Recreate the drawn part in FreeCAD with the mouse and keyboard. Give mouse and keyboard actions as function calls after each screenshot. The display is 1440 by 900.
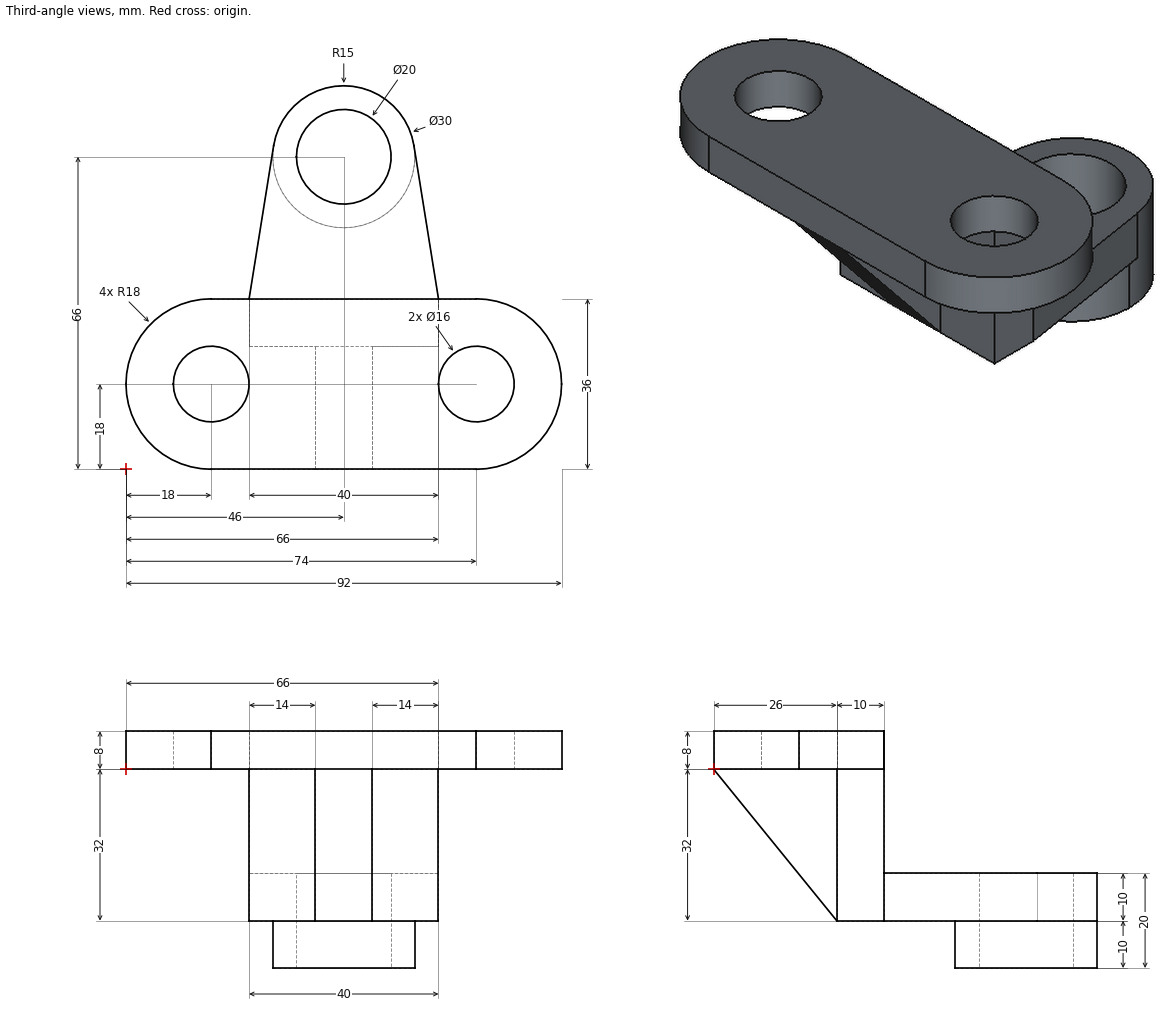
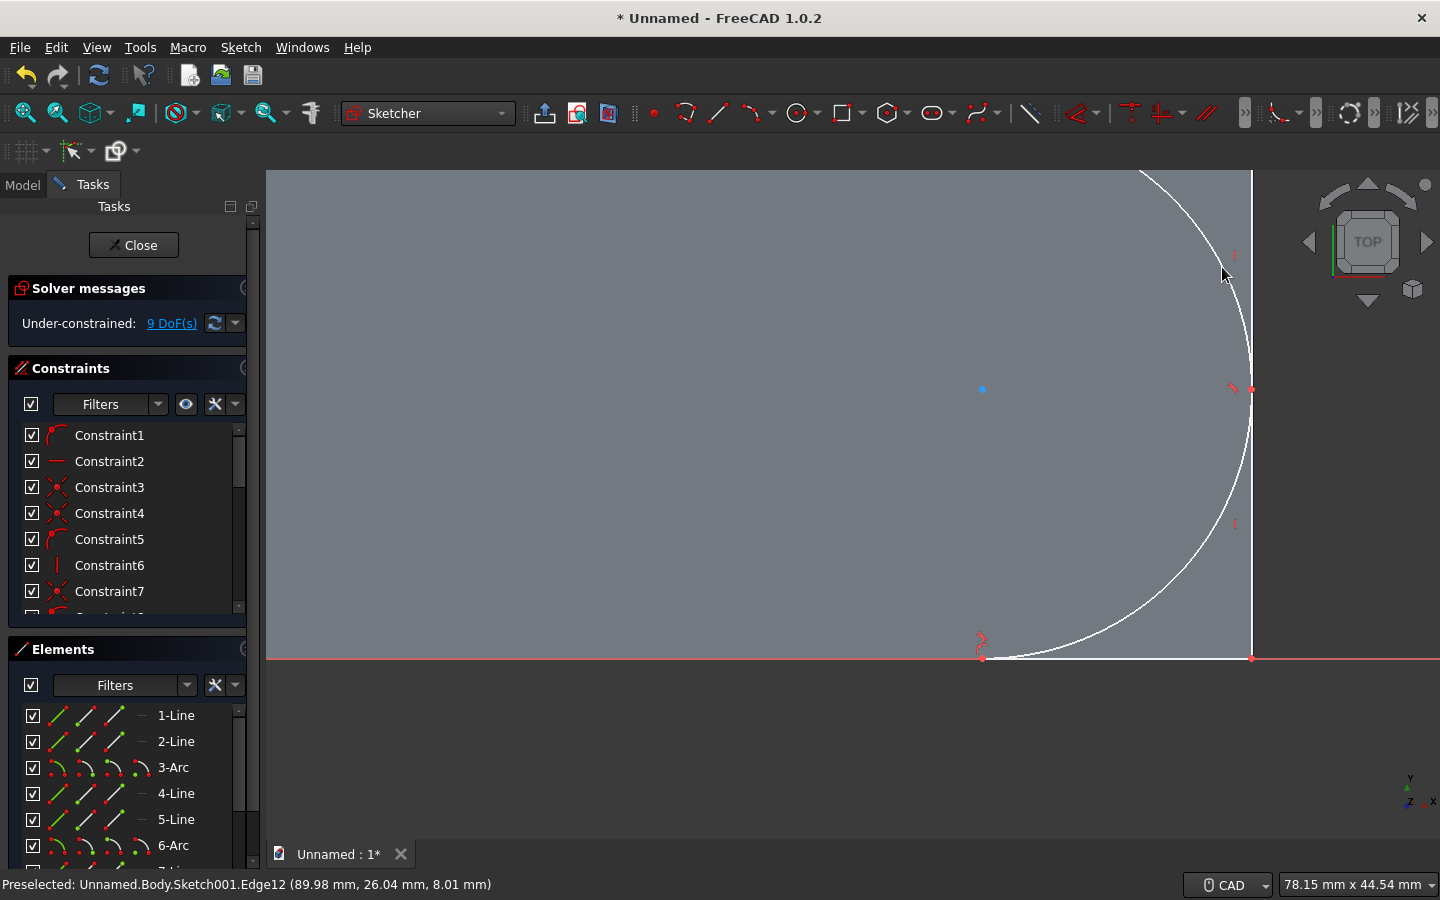
scroll(1055, 646, down, 3)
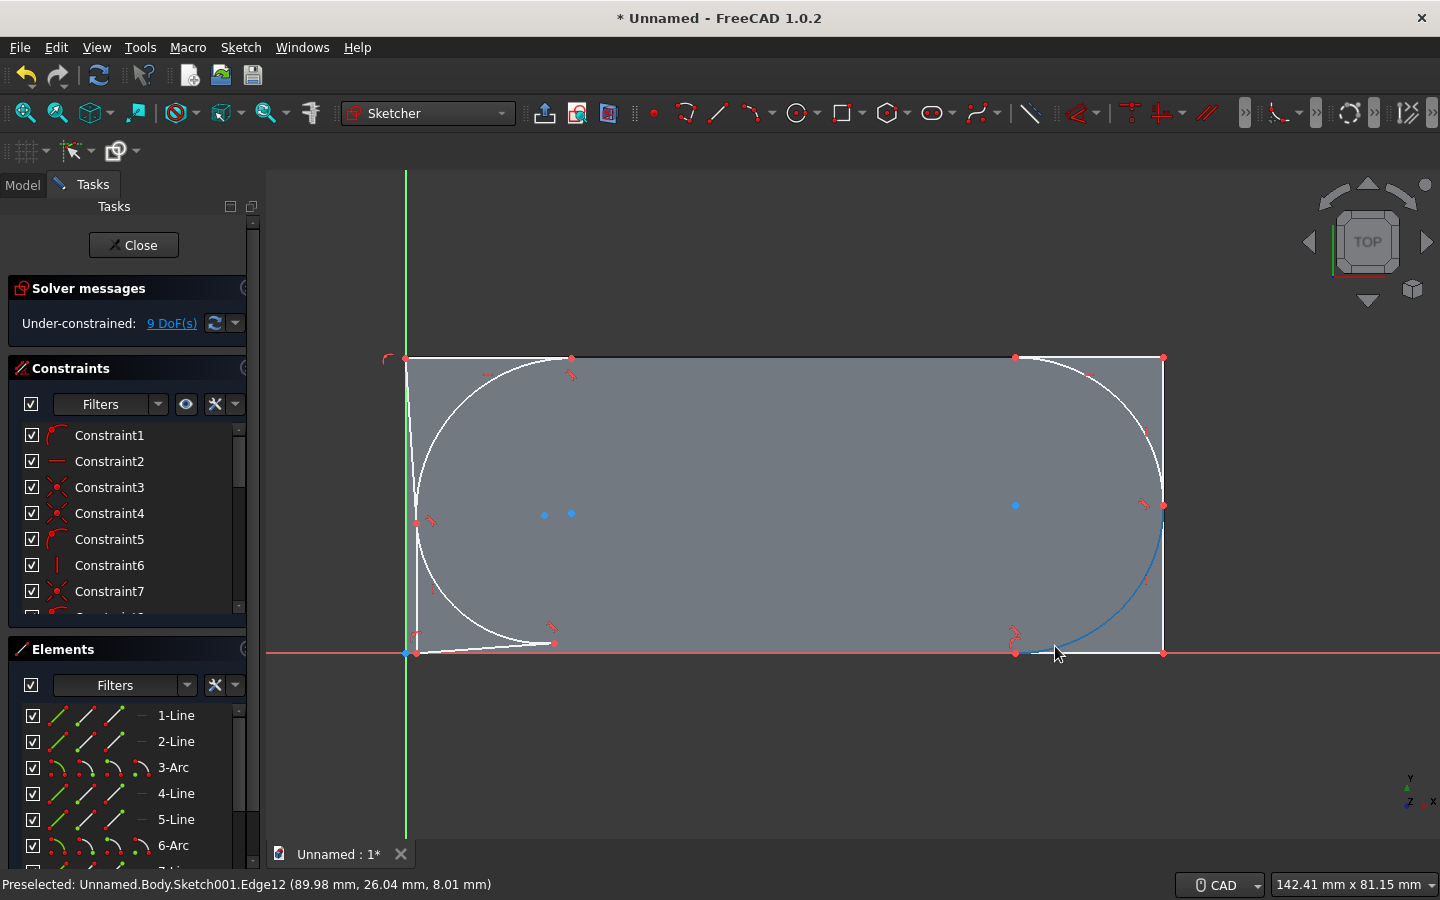
click(1119, 357)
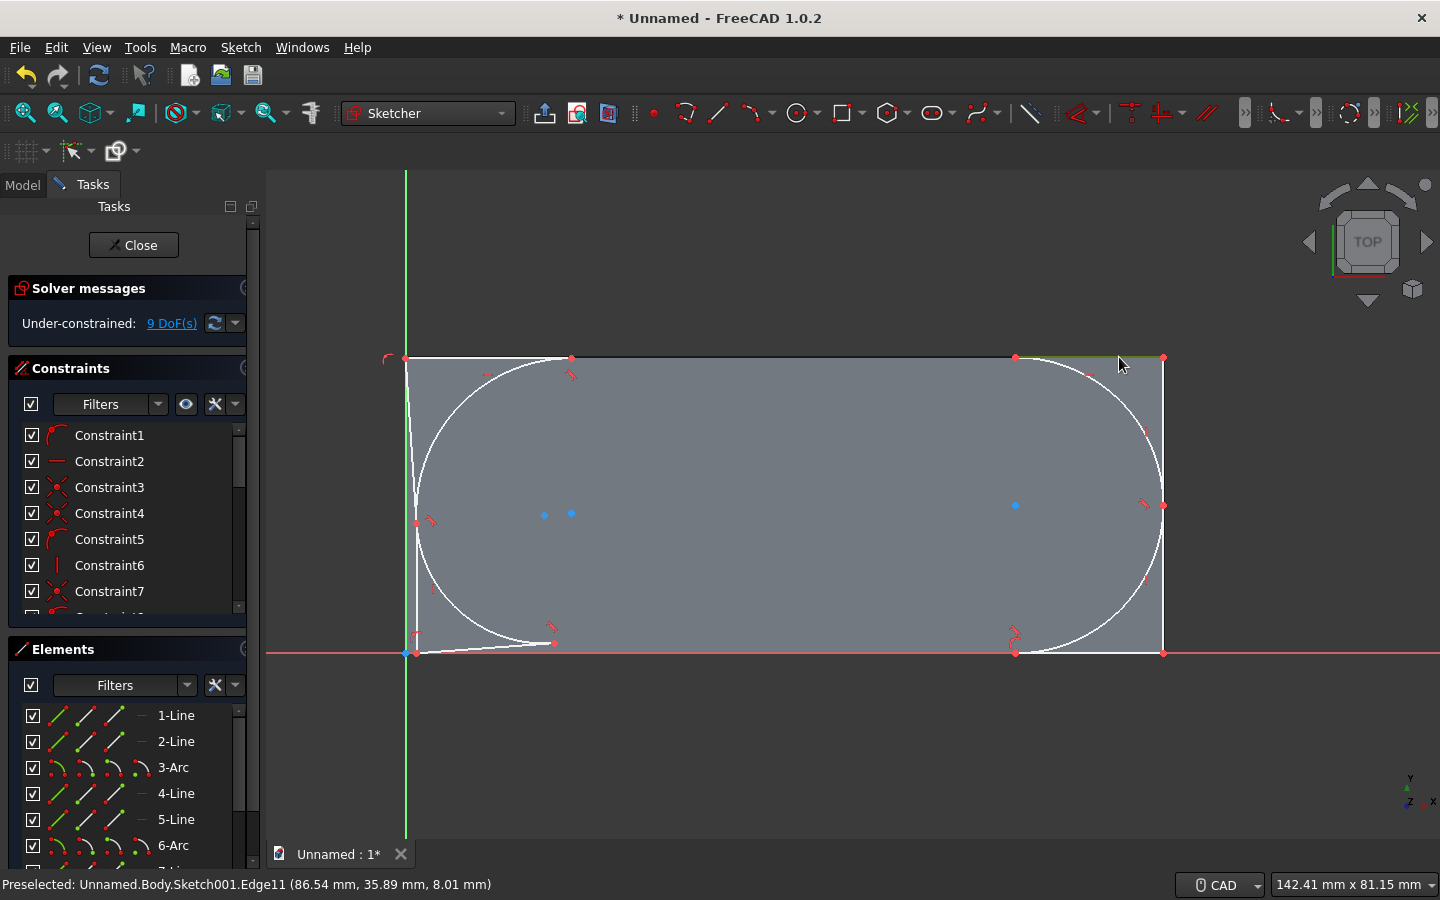
click(1147, 438)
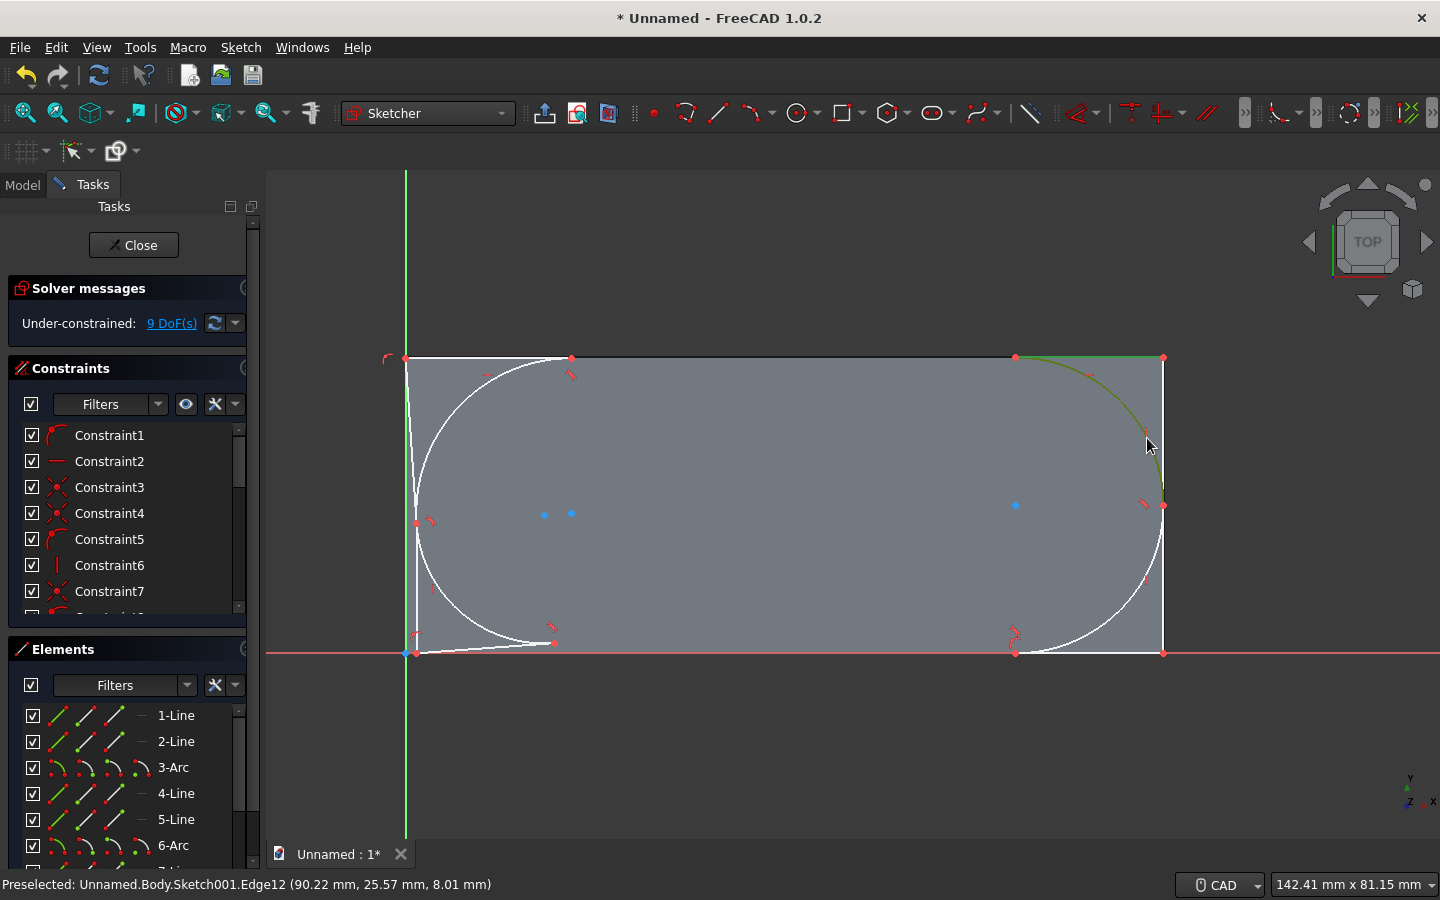
key(t)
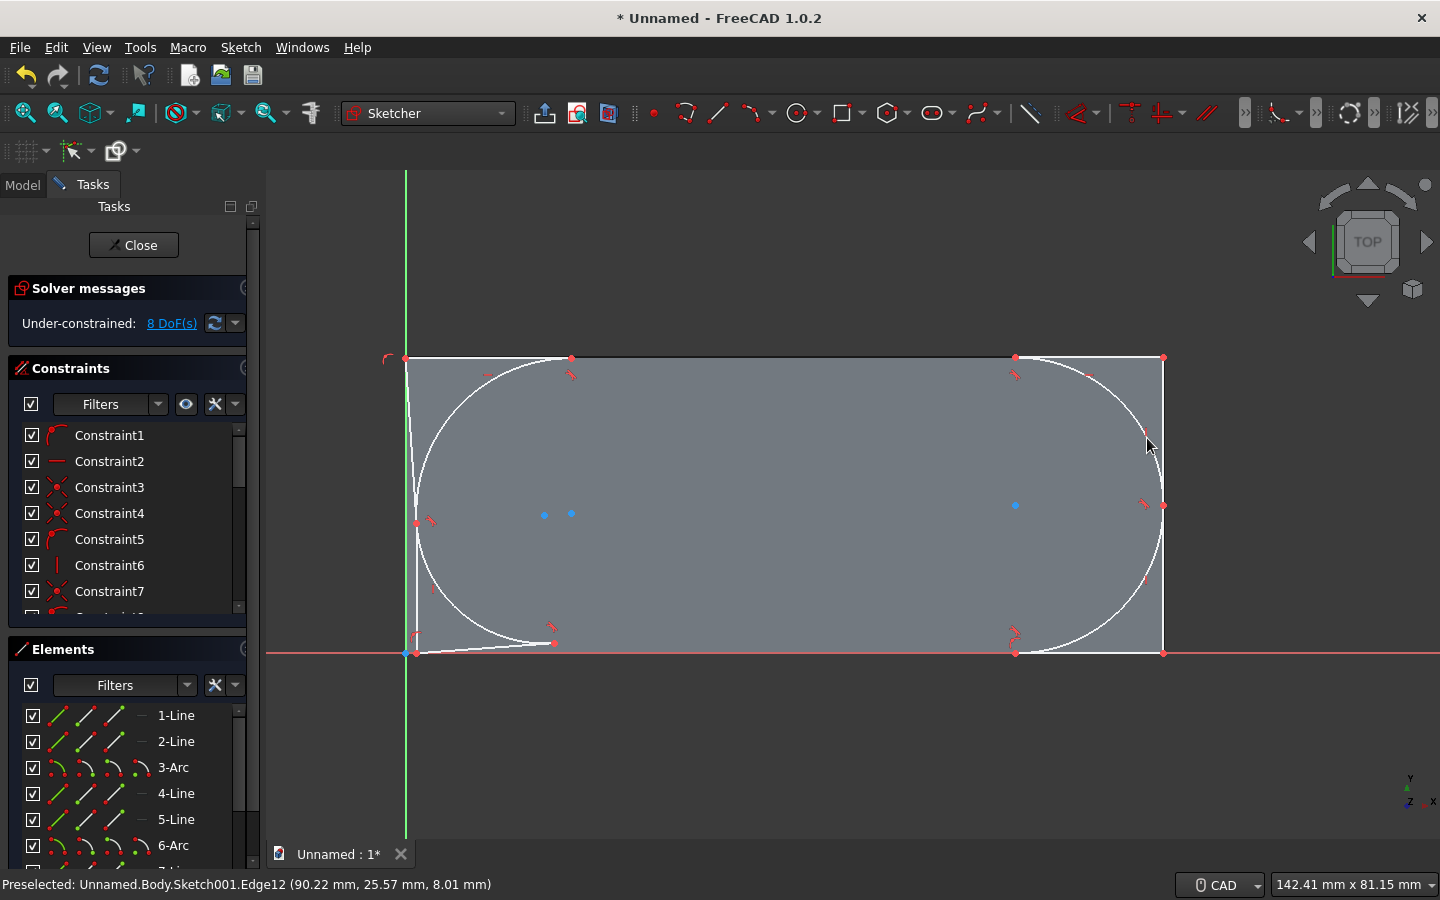
click(409, 408)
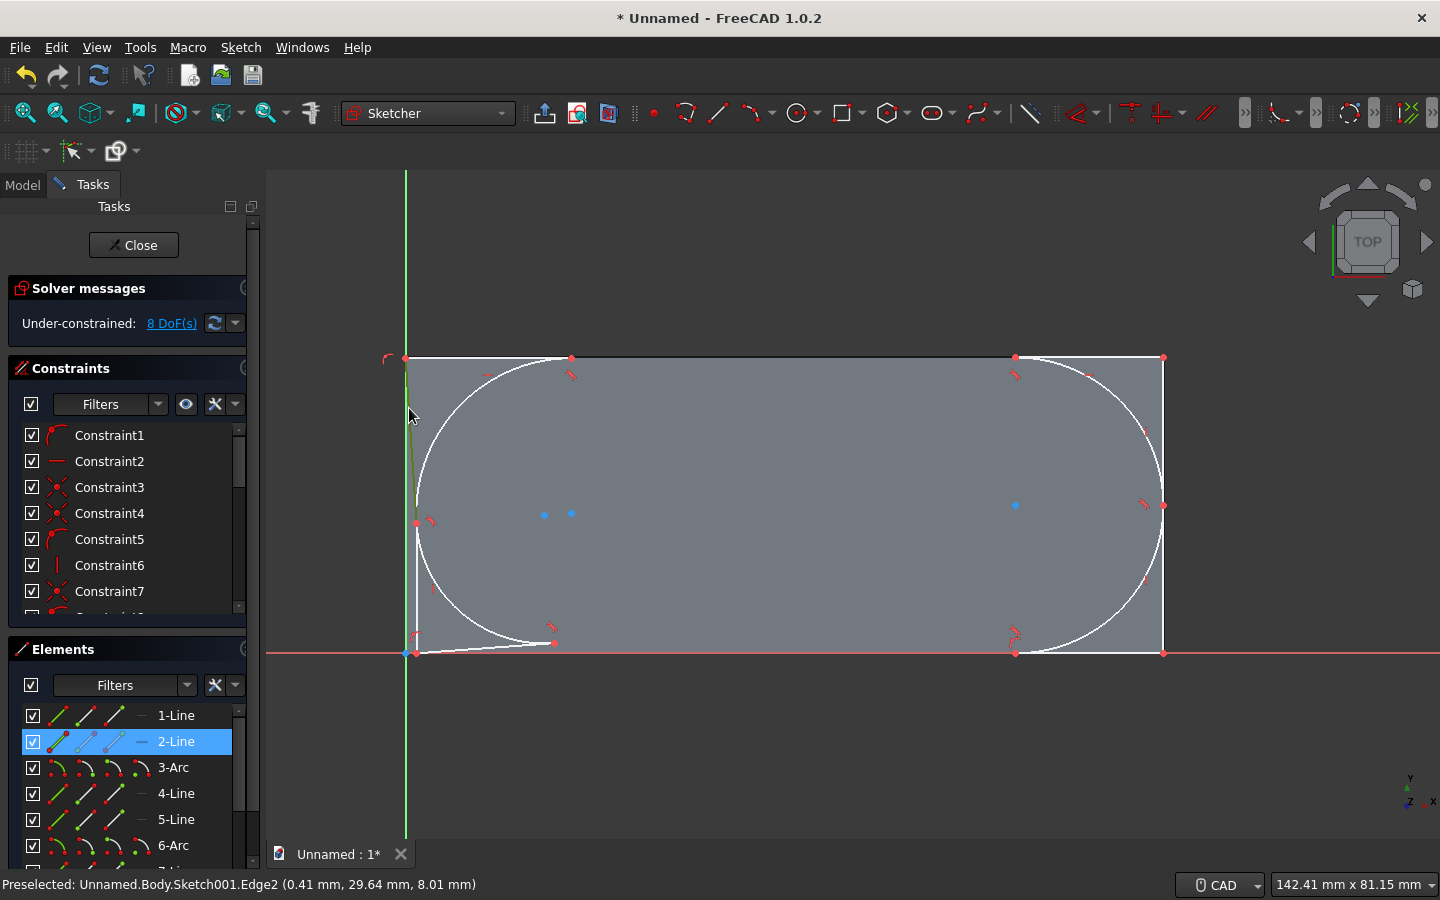
click(1184, 114)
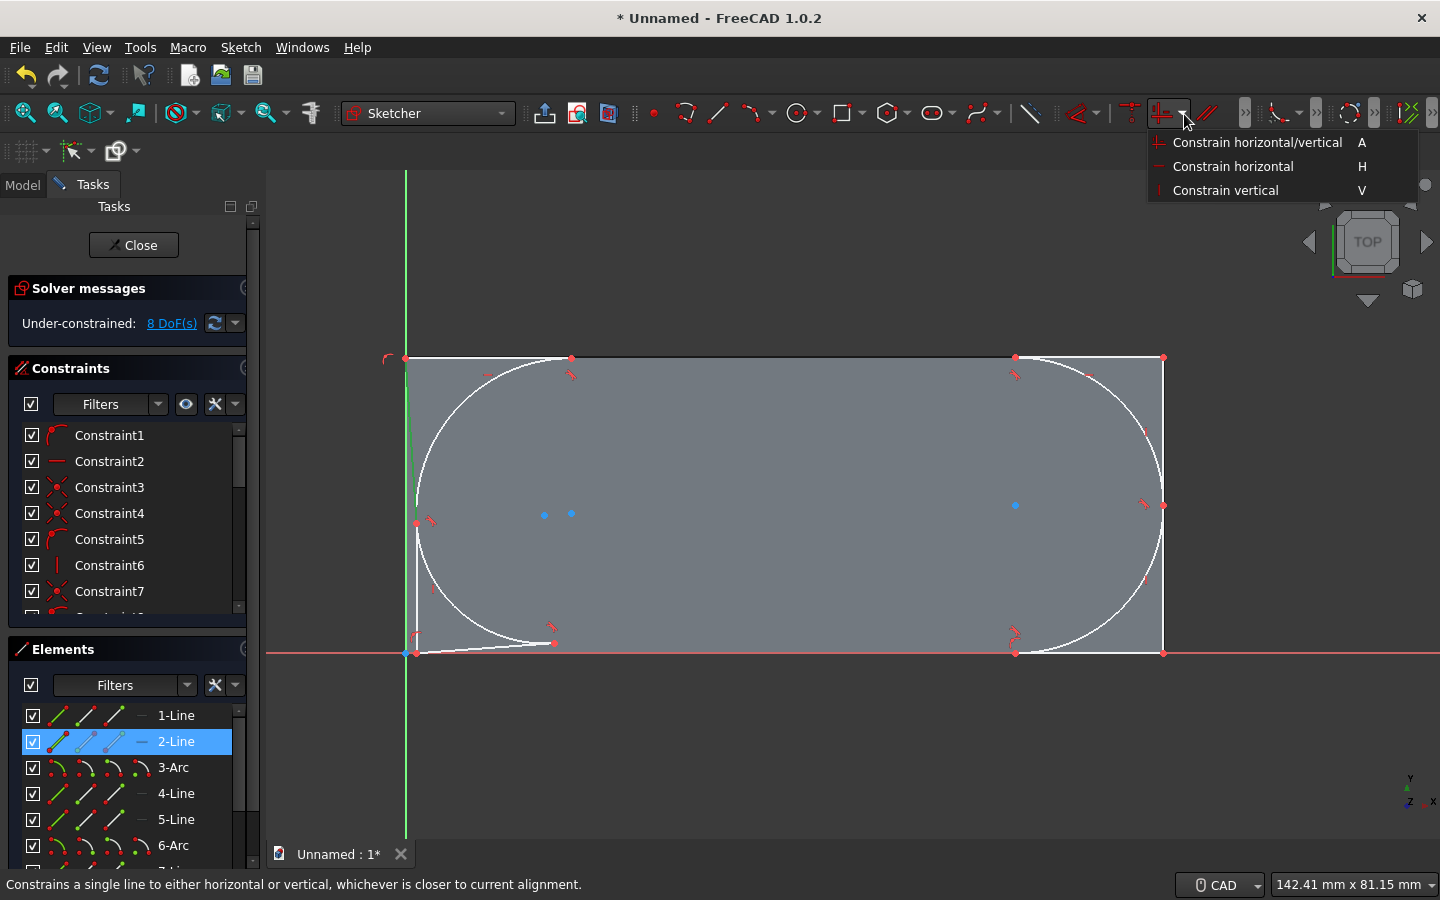
click(1283, 190)